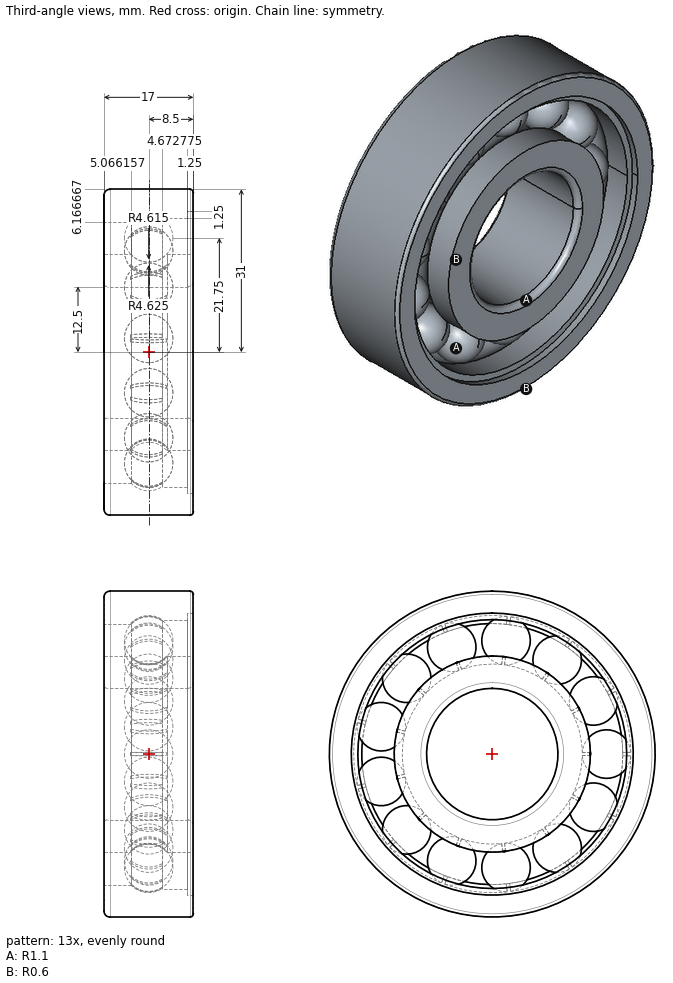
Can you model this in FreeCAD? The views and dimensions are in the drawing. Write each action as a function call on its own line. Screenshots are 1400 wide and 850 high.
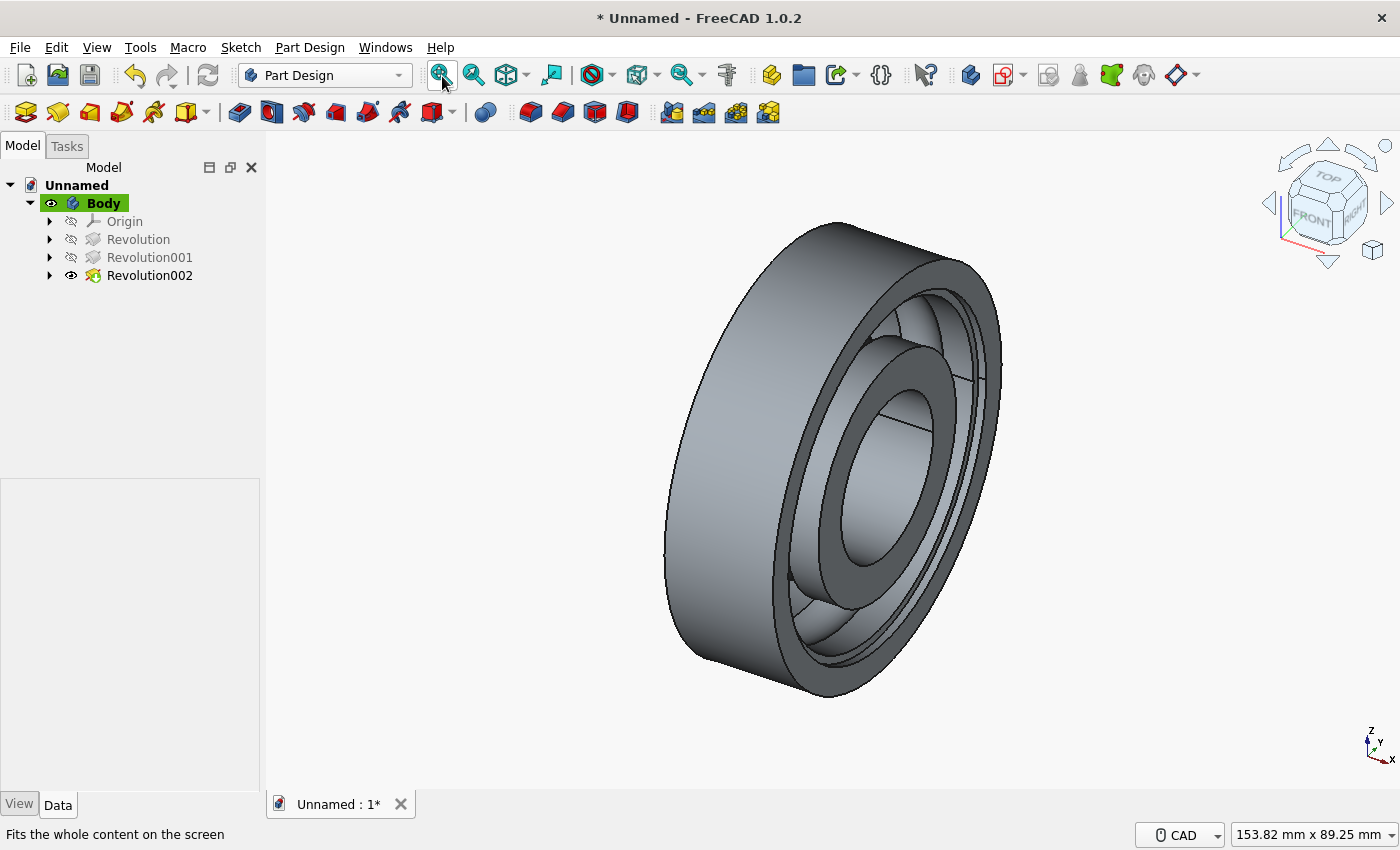
click(116, 239)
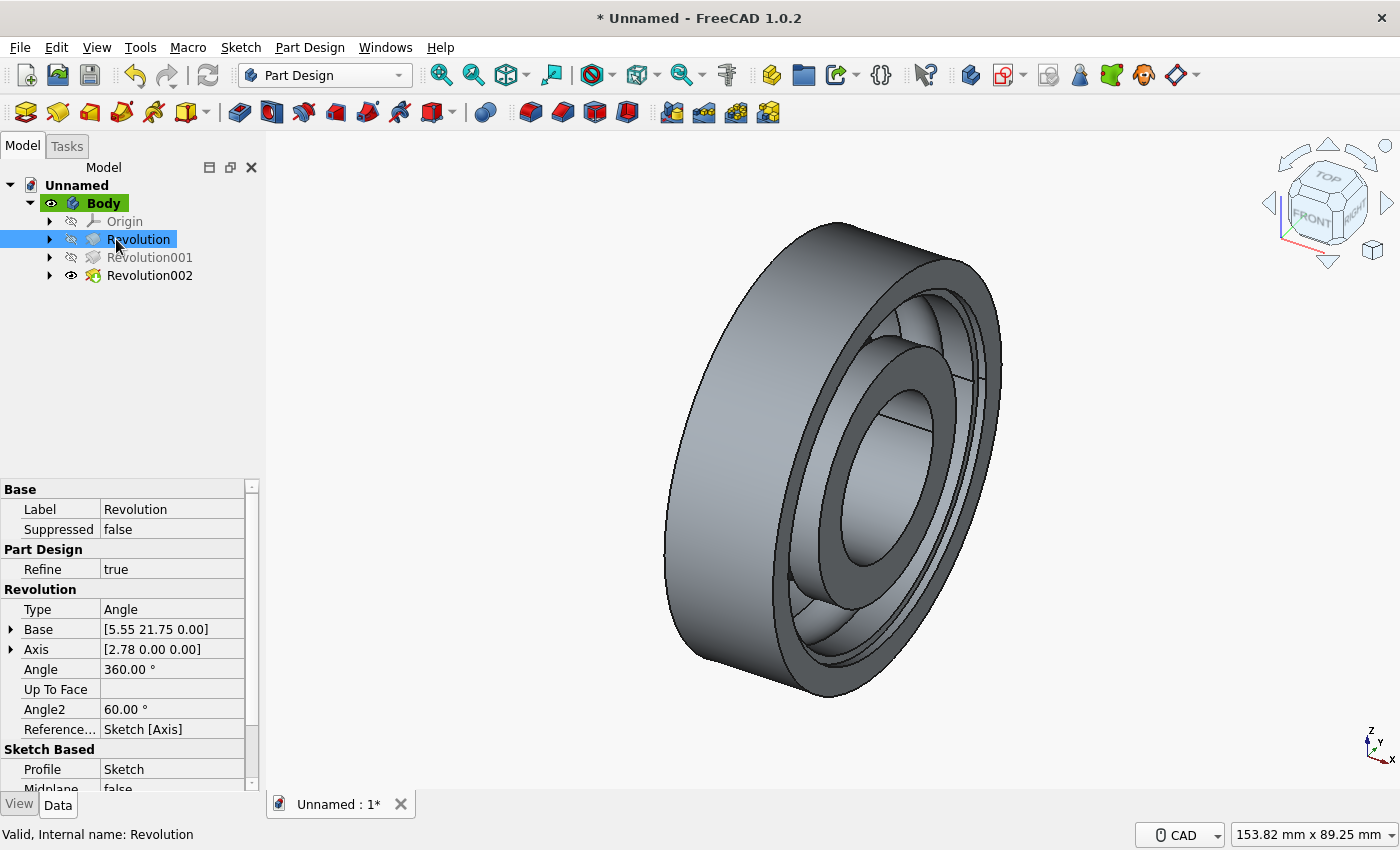
click(736, 112)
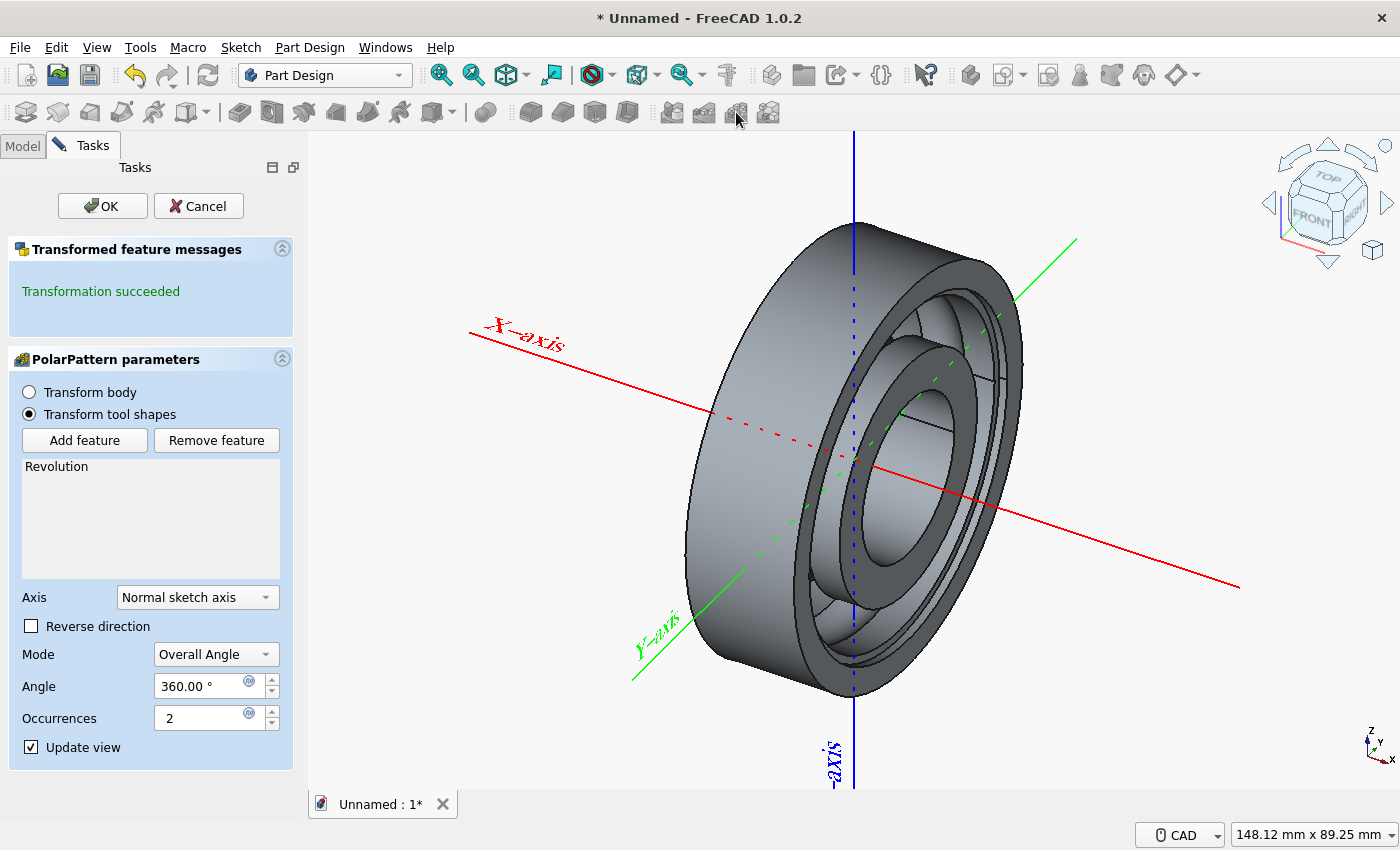
click(198, 598)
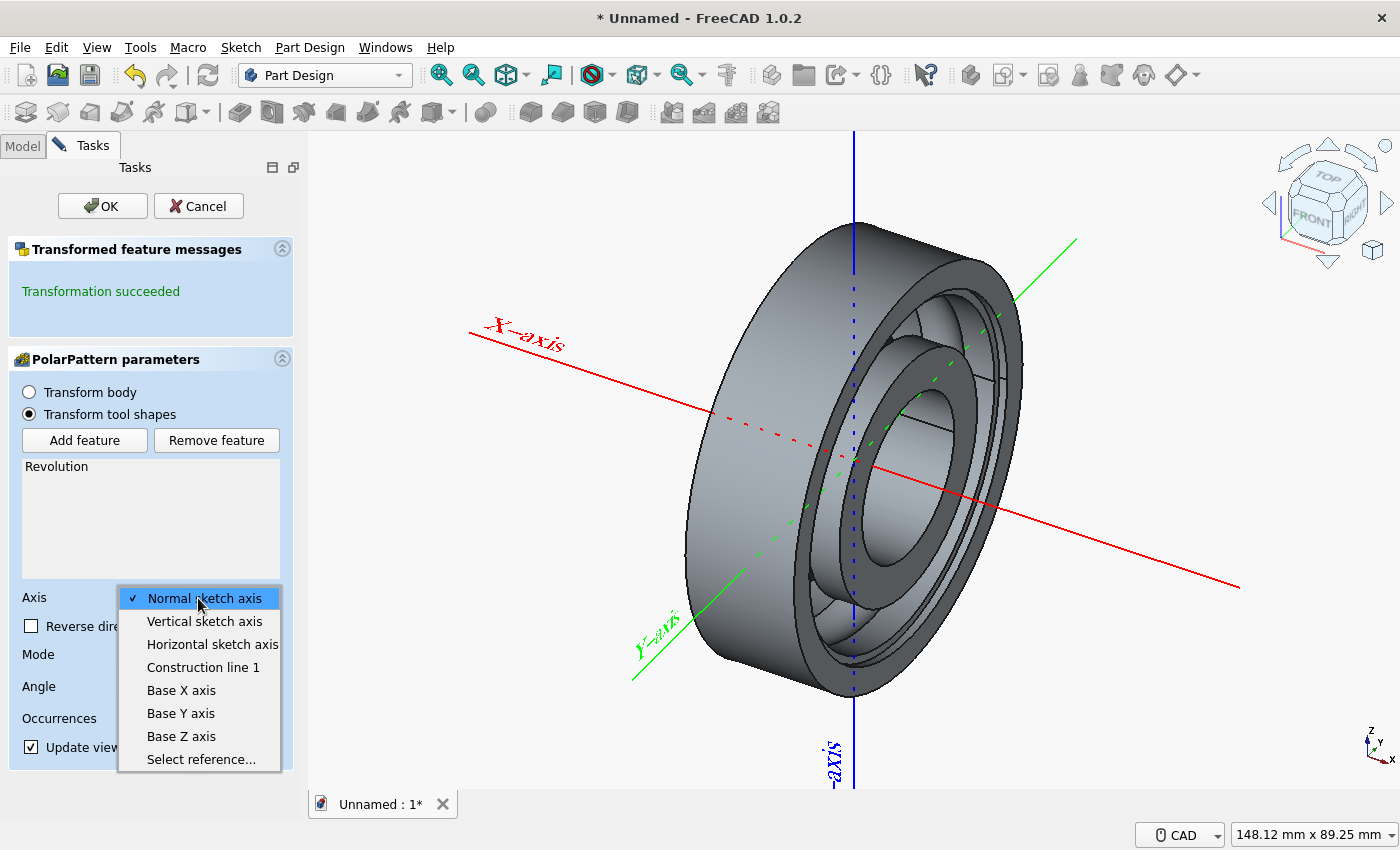
click(198, 690)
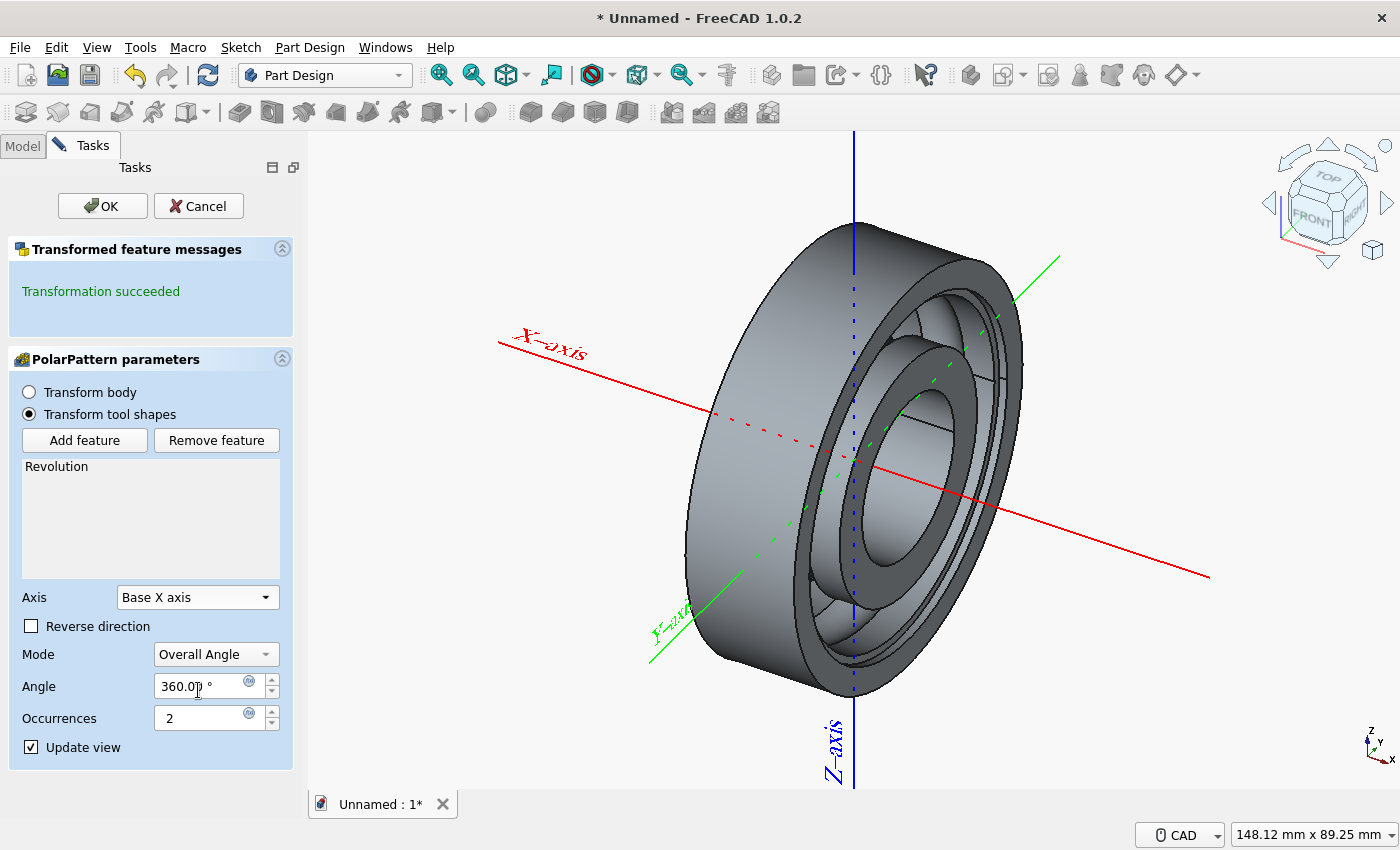
triple_click(209, 718)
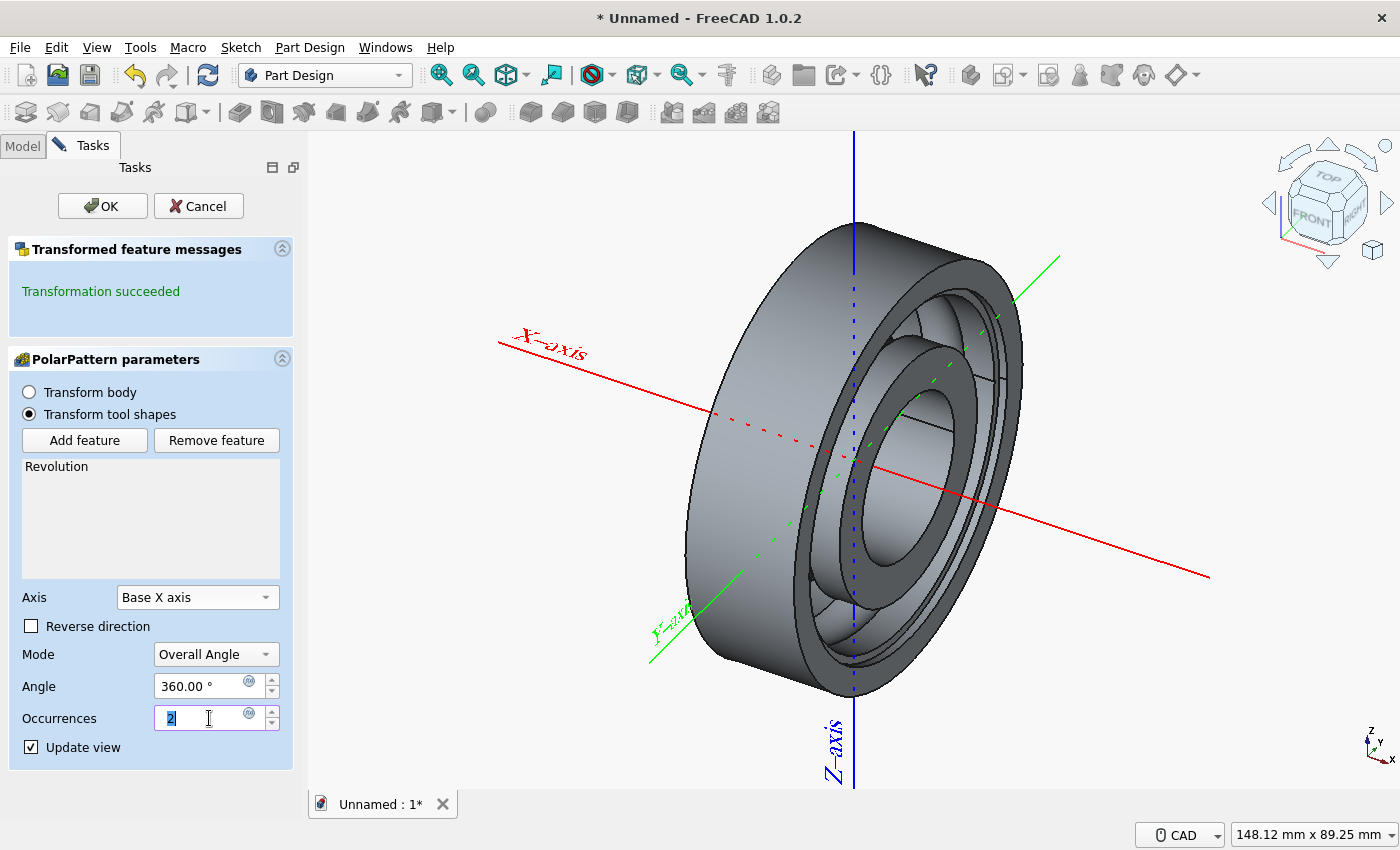
text(13)
key(Tab)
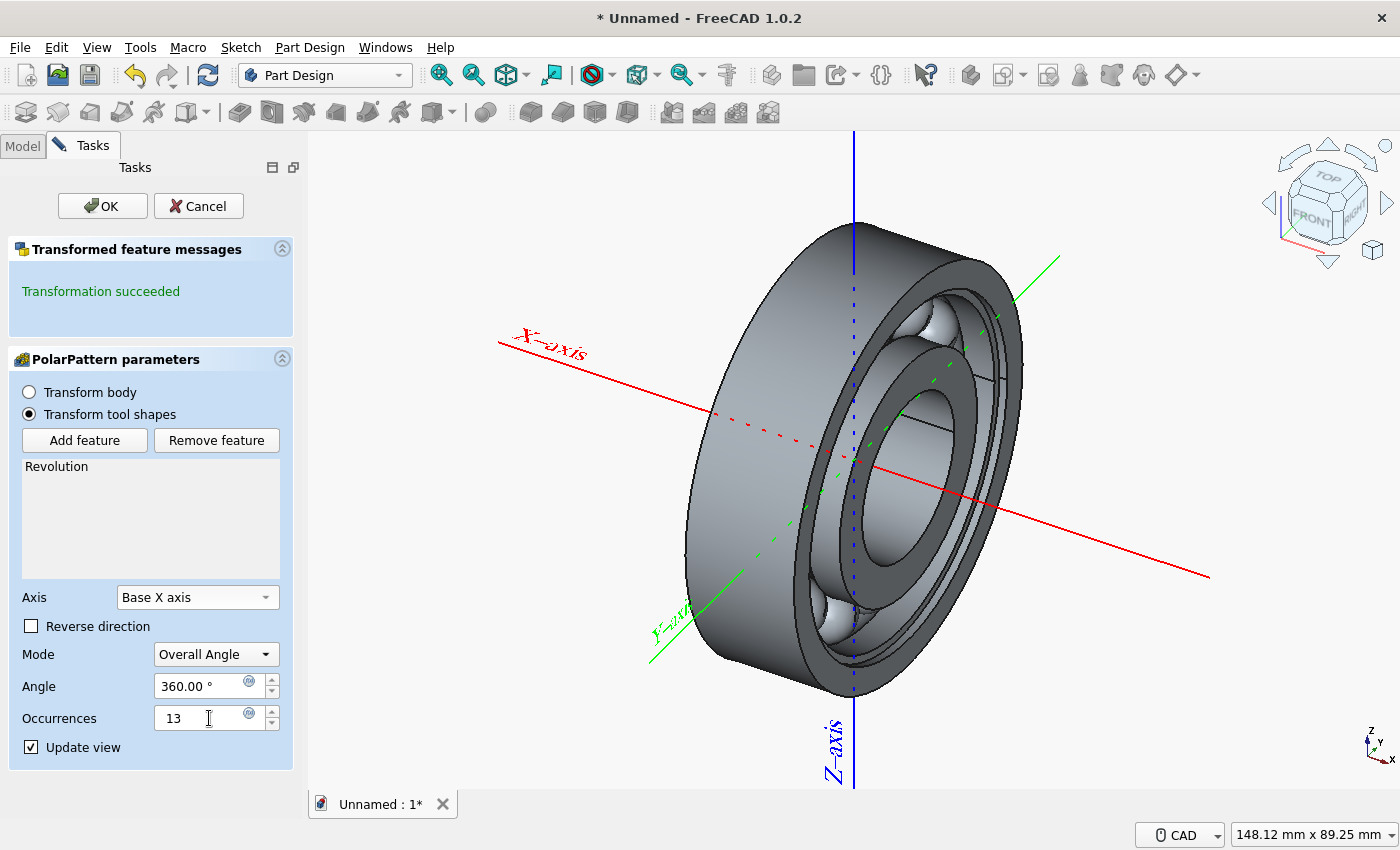
click(103, 206)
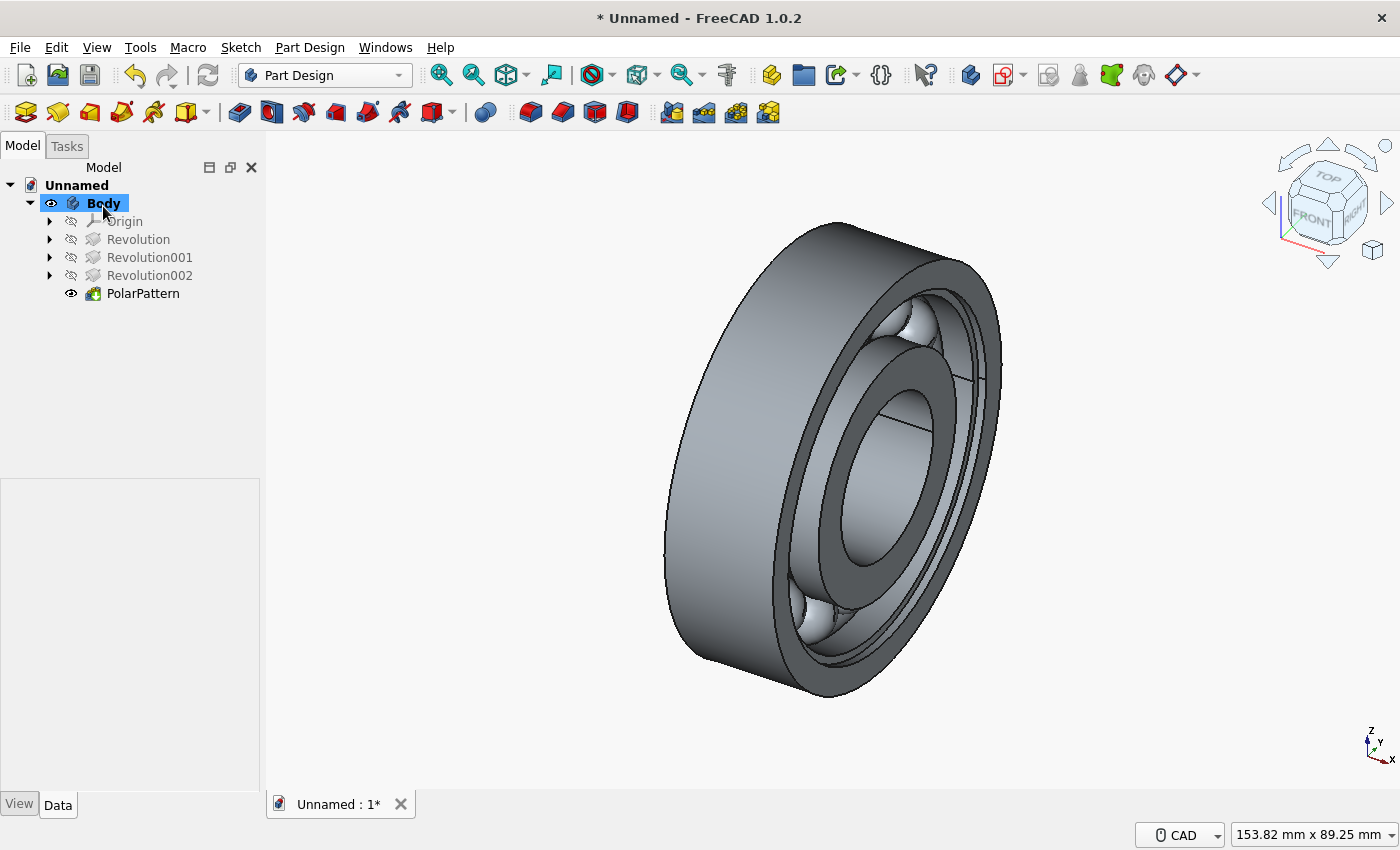
click(873, 563)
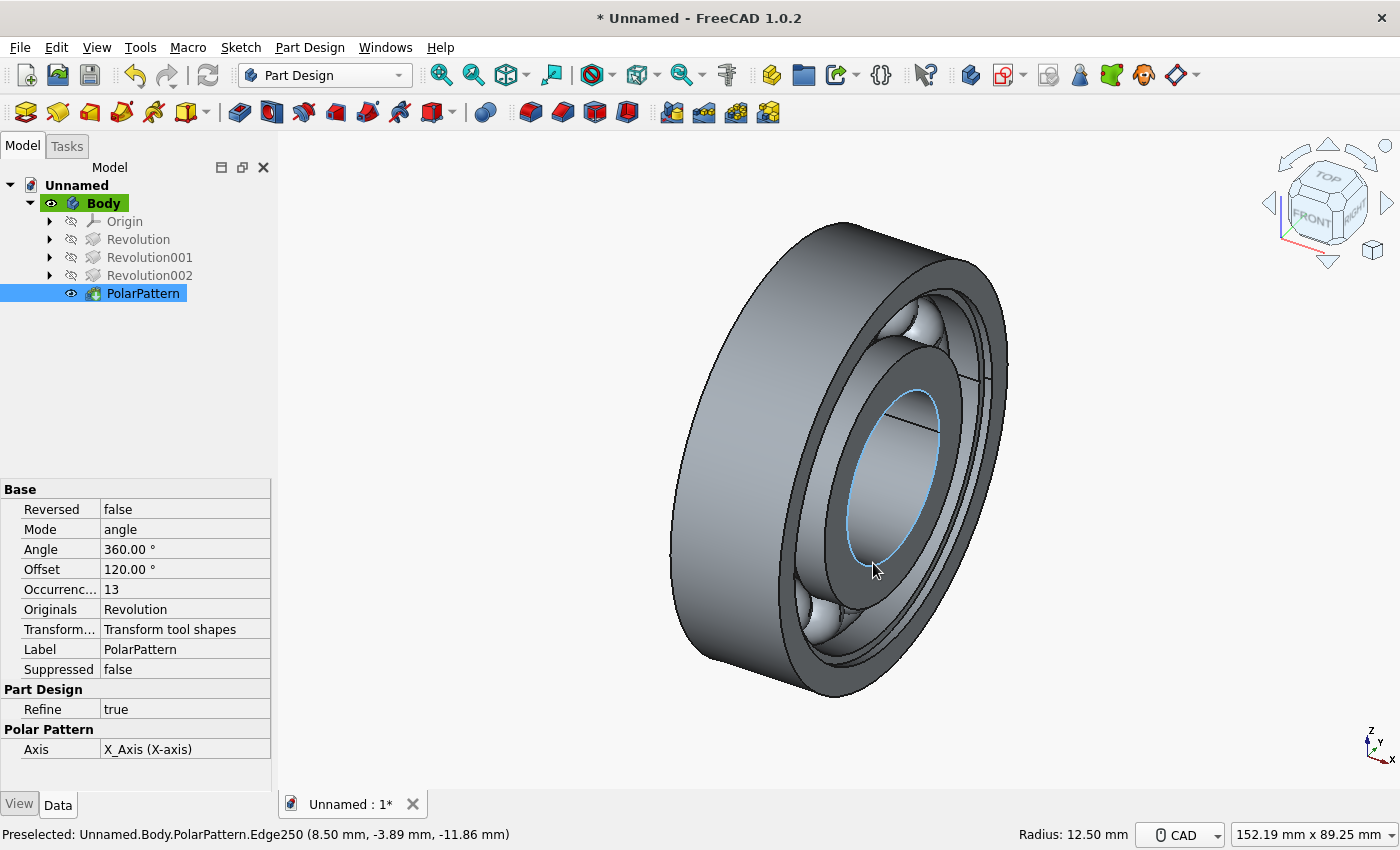
key(0)